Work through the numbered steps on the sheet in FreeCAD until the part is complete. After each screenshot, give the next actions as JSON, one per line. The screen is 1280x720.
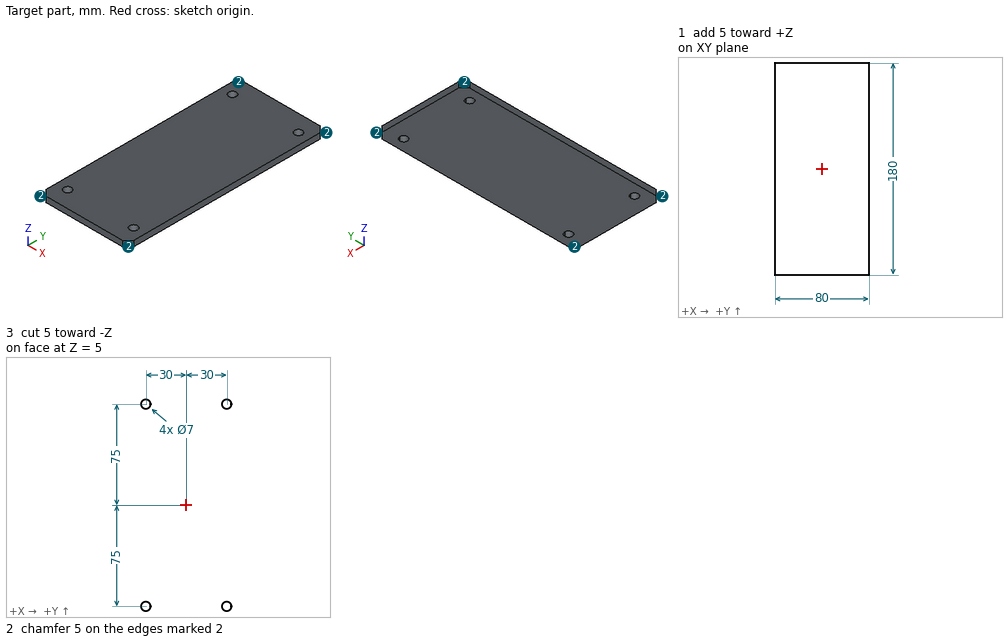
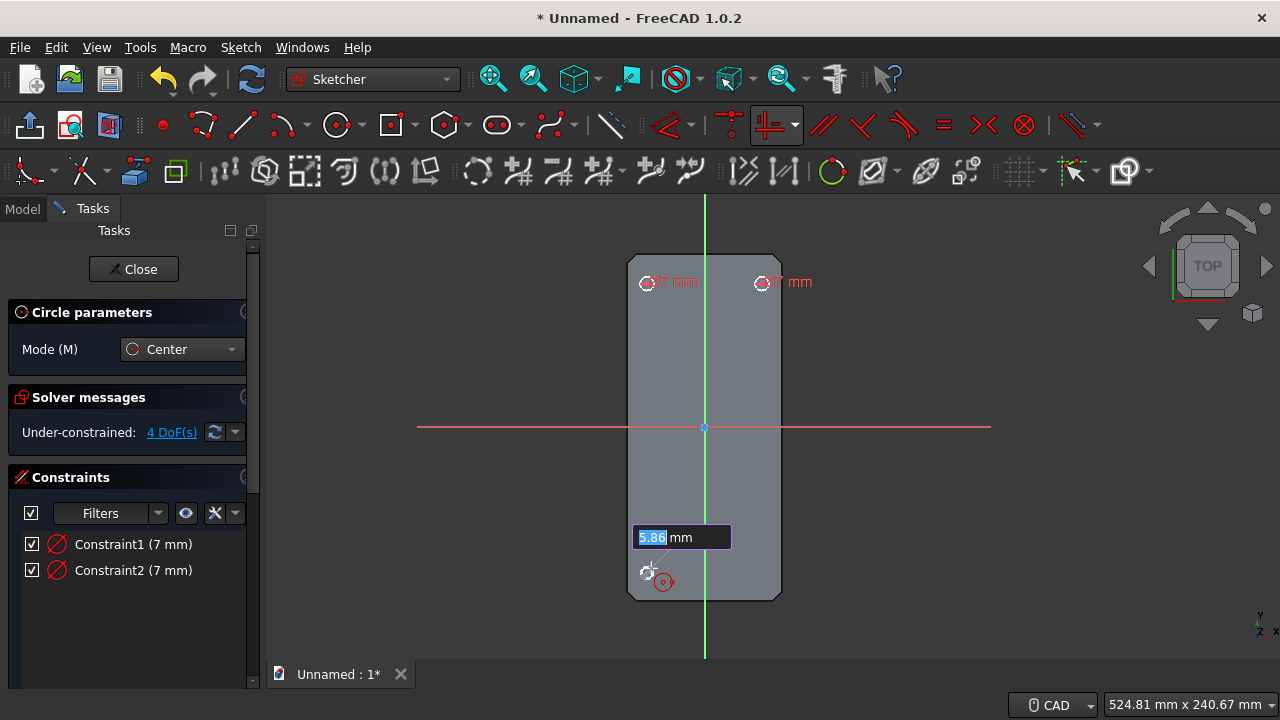
{"action": "type", "text": "7"}
{"action": "key", "text": "Return"}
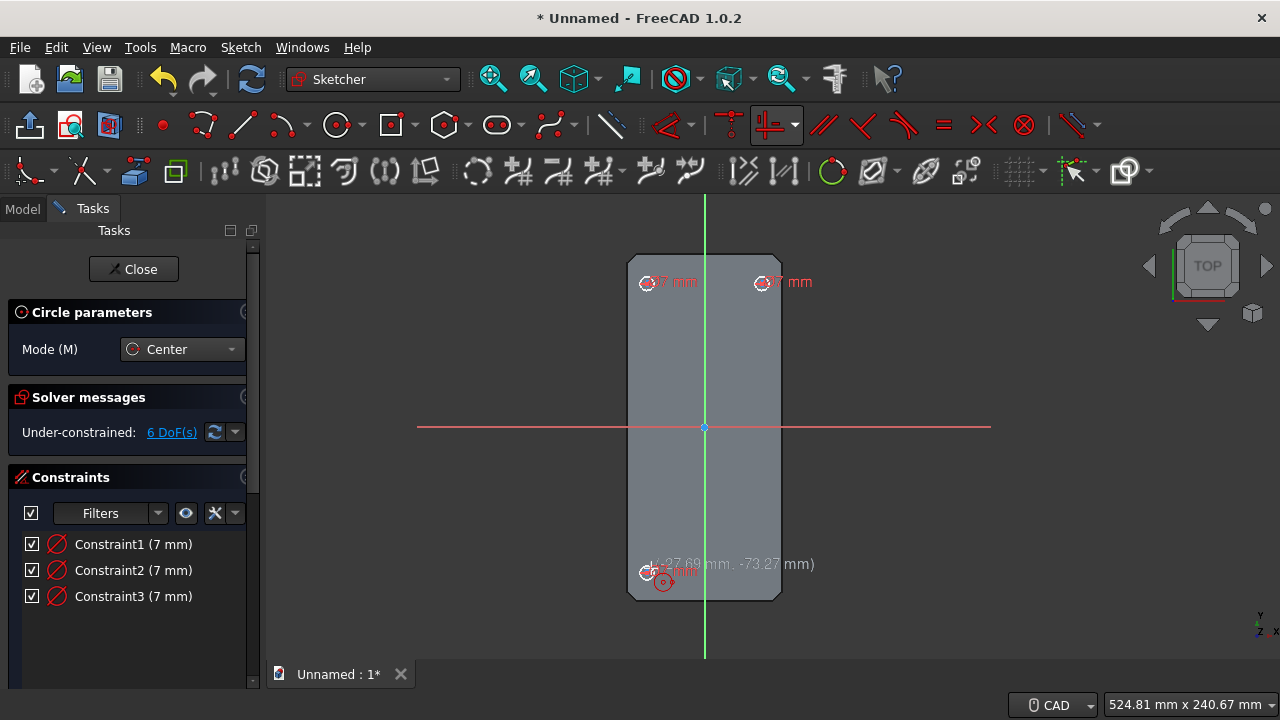
{"action": "scroll", "coordinate": [762, 572], "scroll_direction": "up", "scroll_amount": 7}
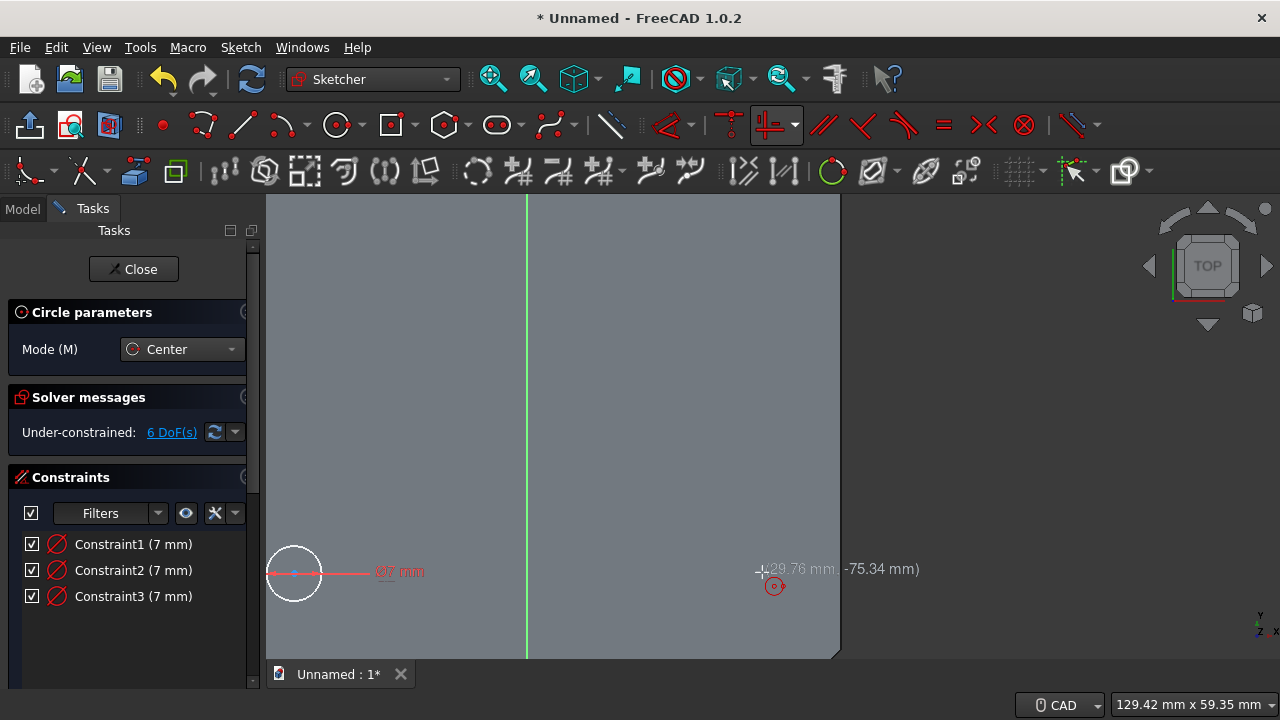
{"action": "scroll", "coordinate": [762, 572], "scroll_direction": "down", "scroll_amount": 7}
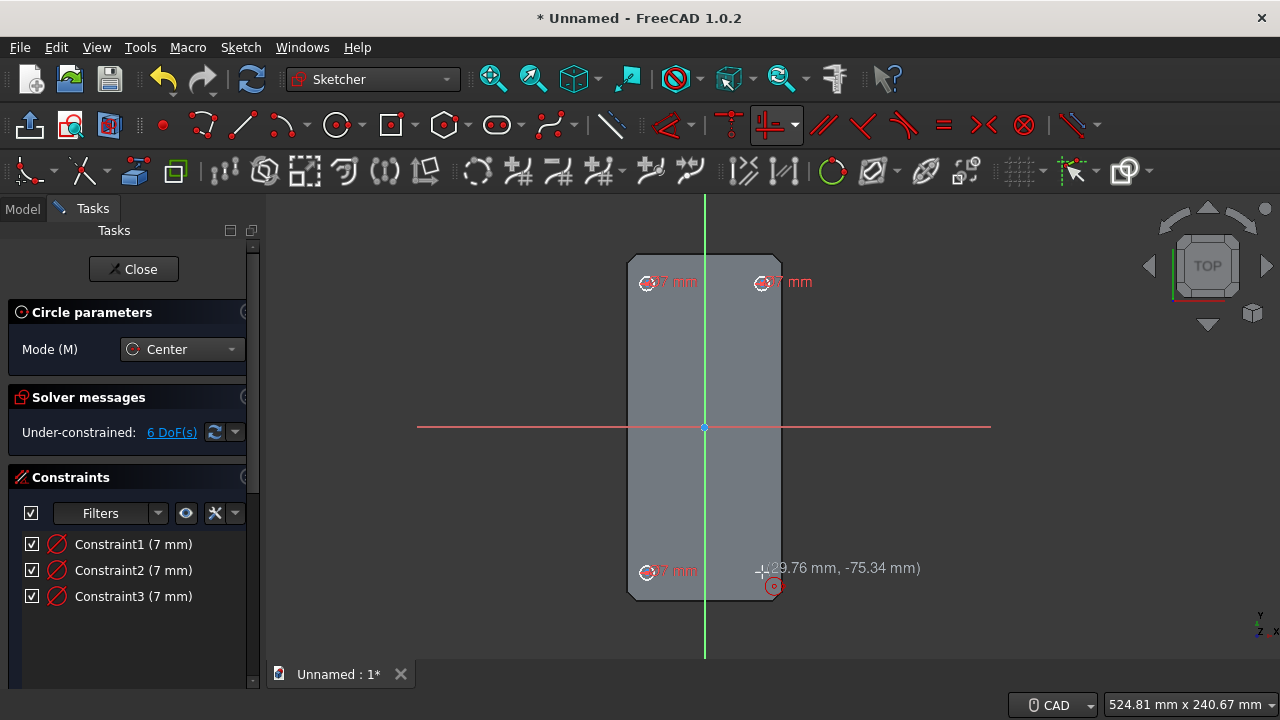
{"action": "left_click", "coordinate": [762, 572]}
{"action": "mouse_move", "coordinate": [767, 568]}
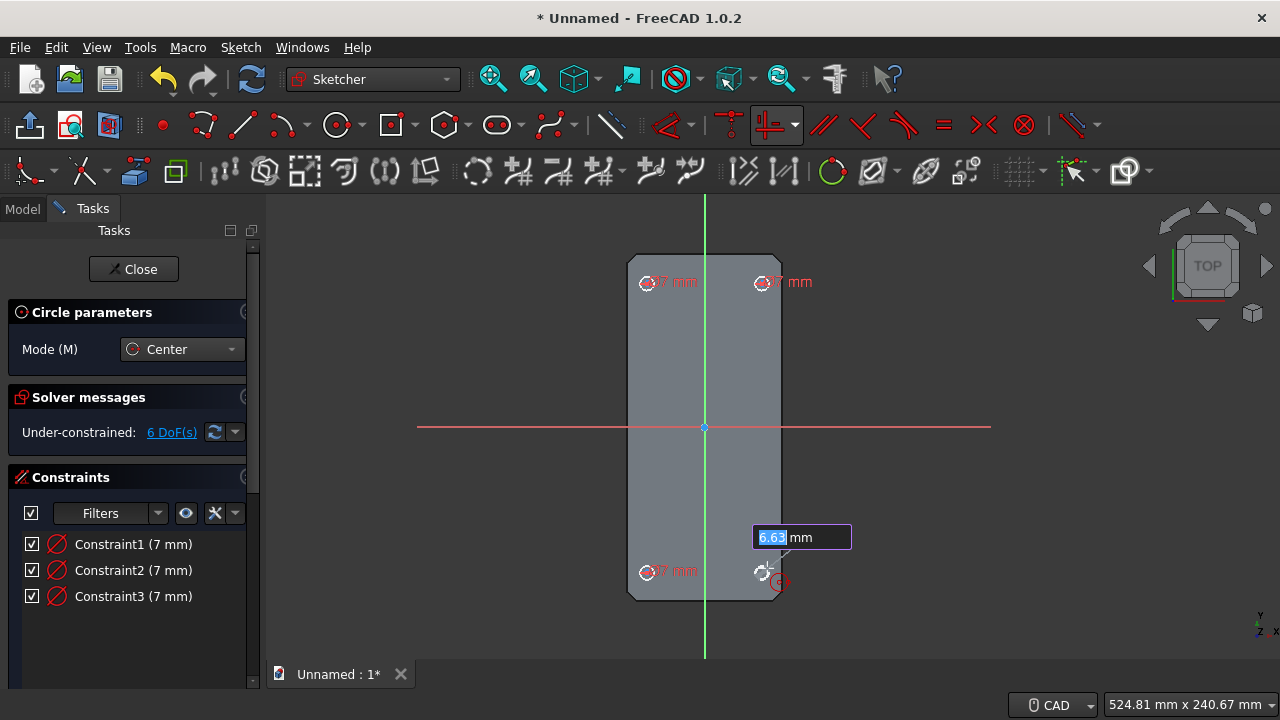
{"action": "type", "text": "7"}
{"action": "key", "text": "Return"}
{"action": "key", "text": "Escape"}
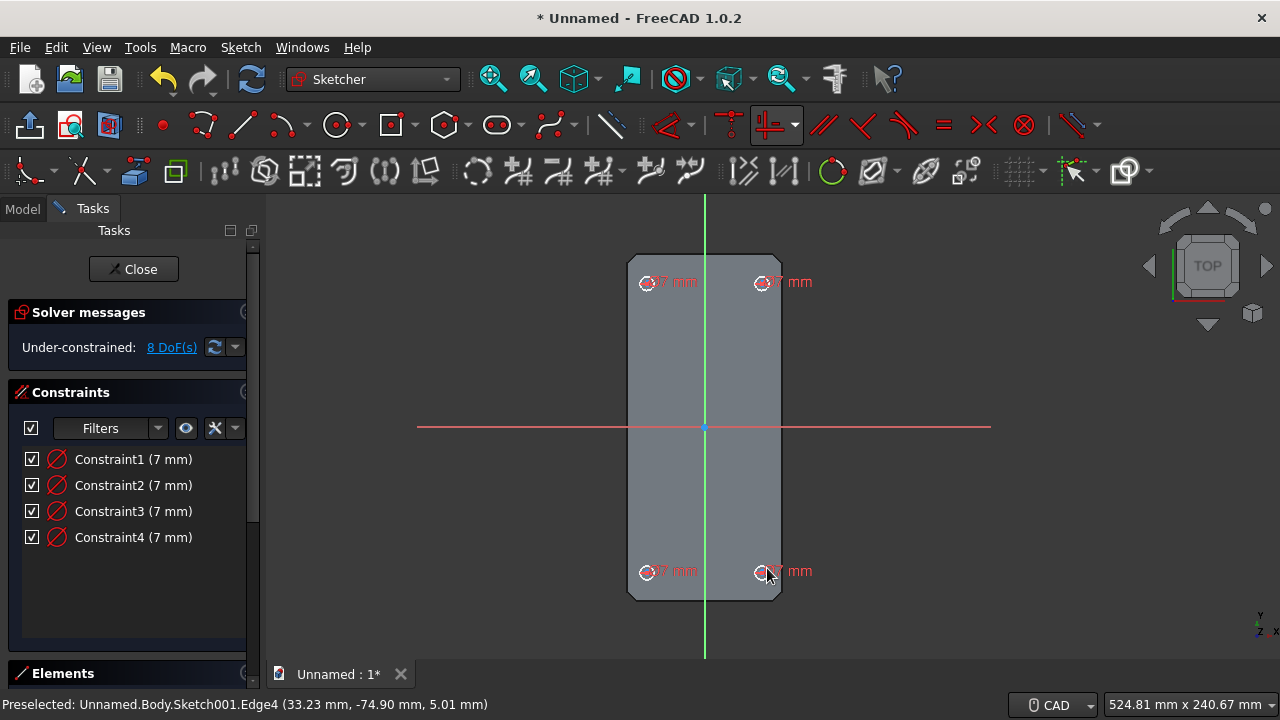
{"action": "left_click", "coordinate": [647, 284]}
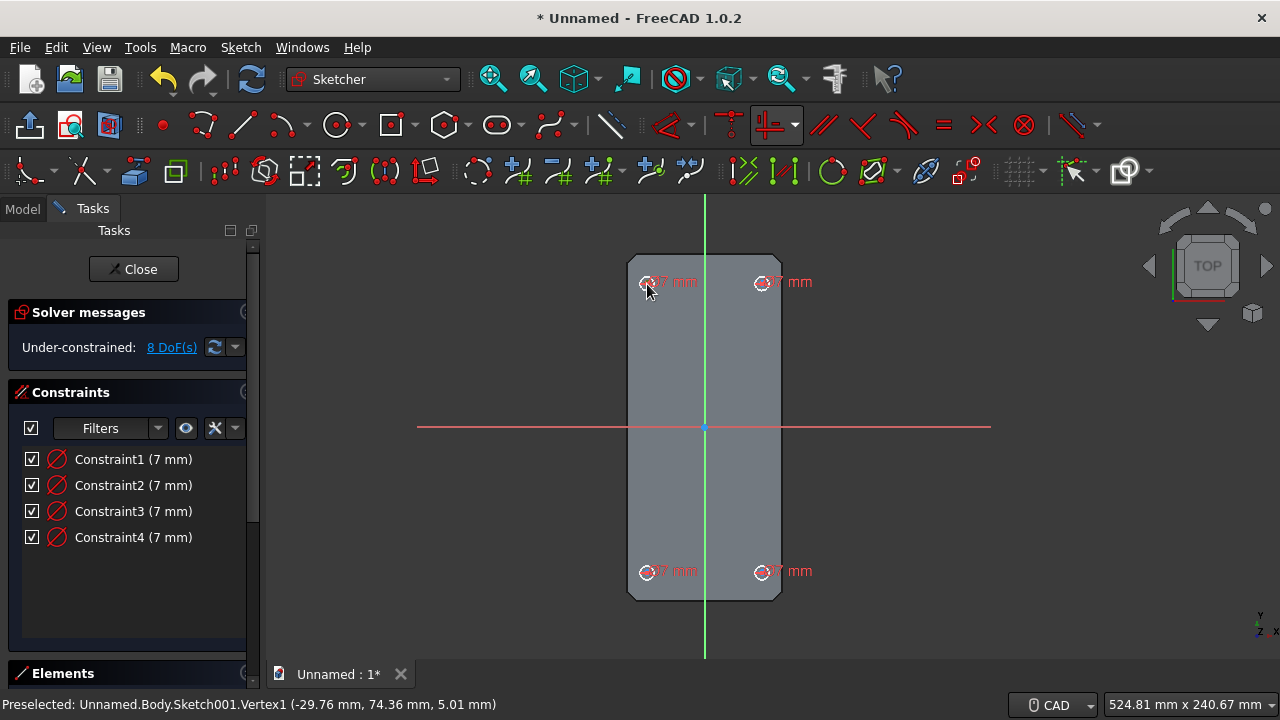
{"action": "left_click", "coordinate": [762, 284]}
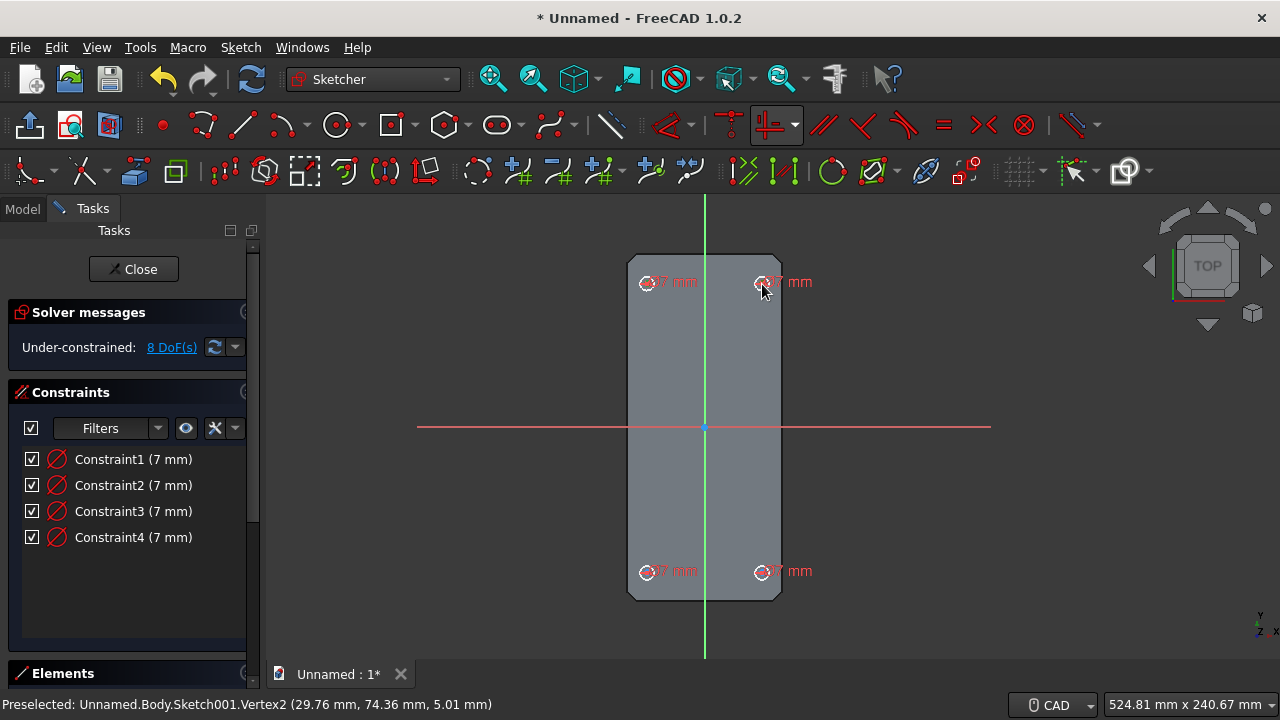
{"action": "left_click", "coordinate": [798, 126]}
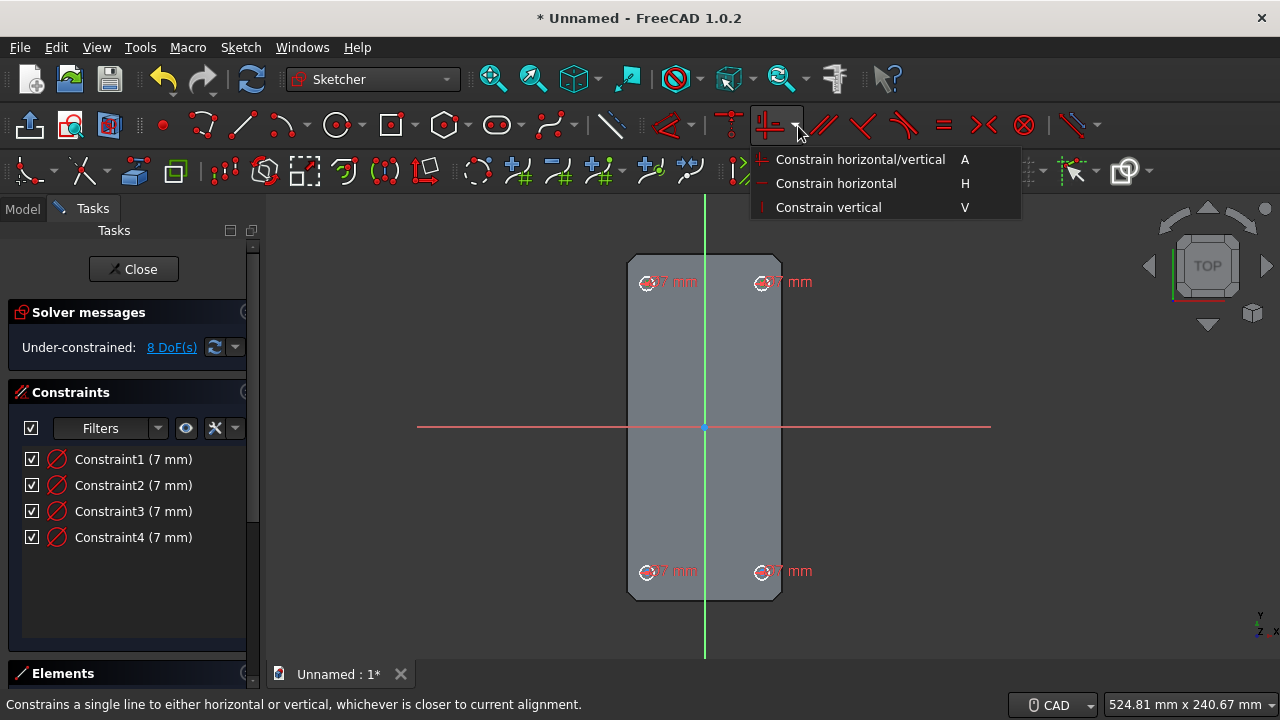
{"action": "left_click", "coordinate": [886, 183]}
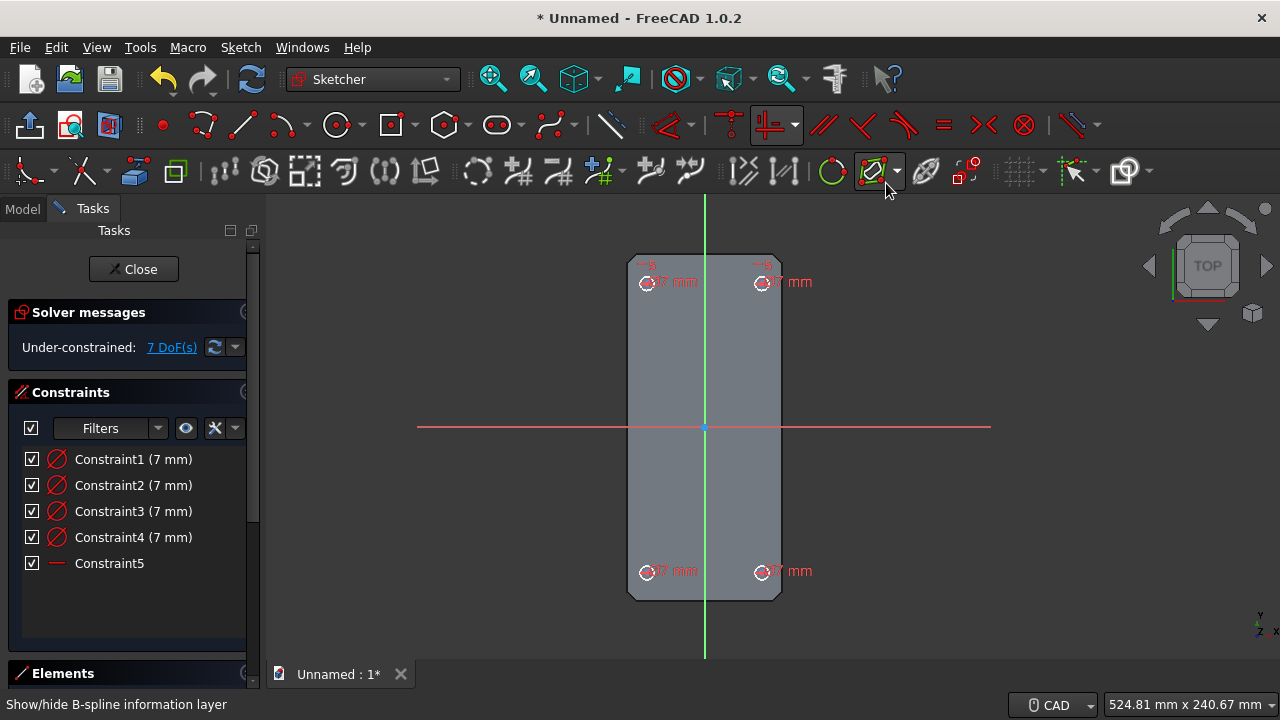
{"action": "left_click", "coordinate": [647, 284]}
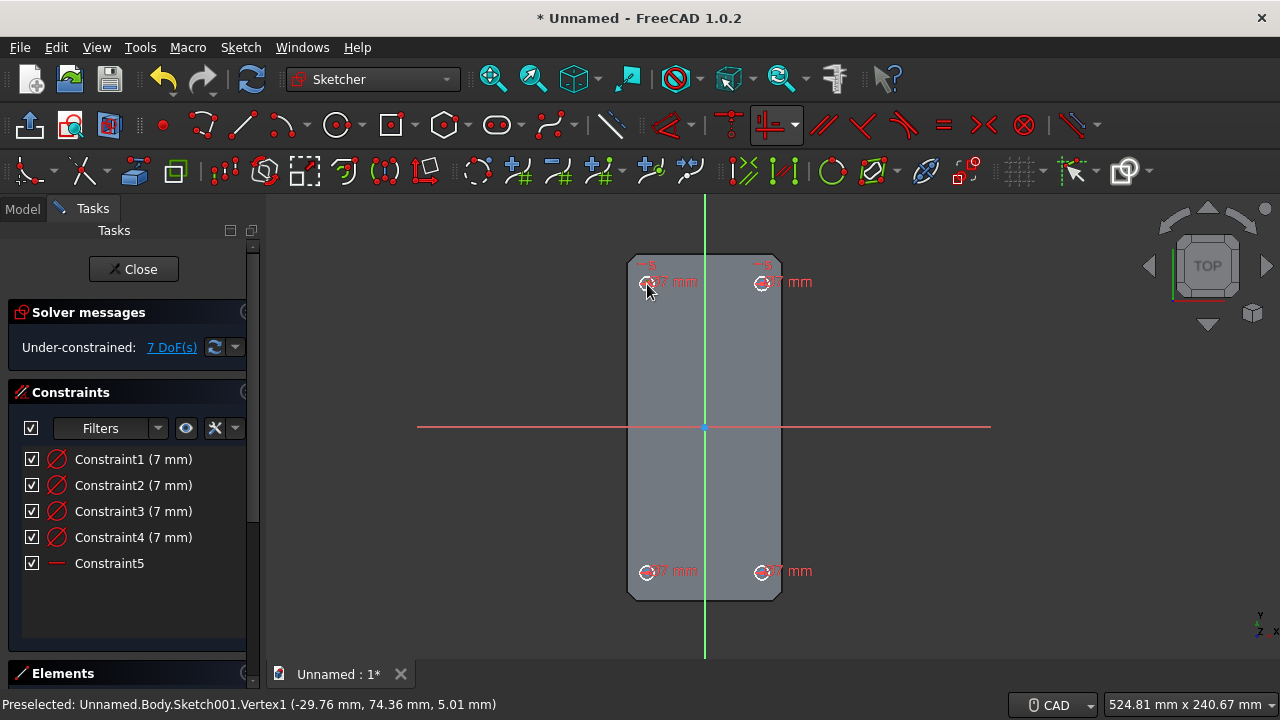
{"action": "left_click", "coordinate": [647, 573]}